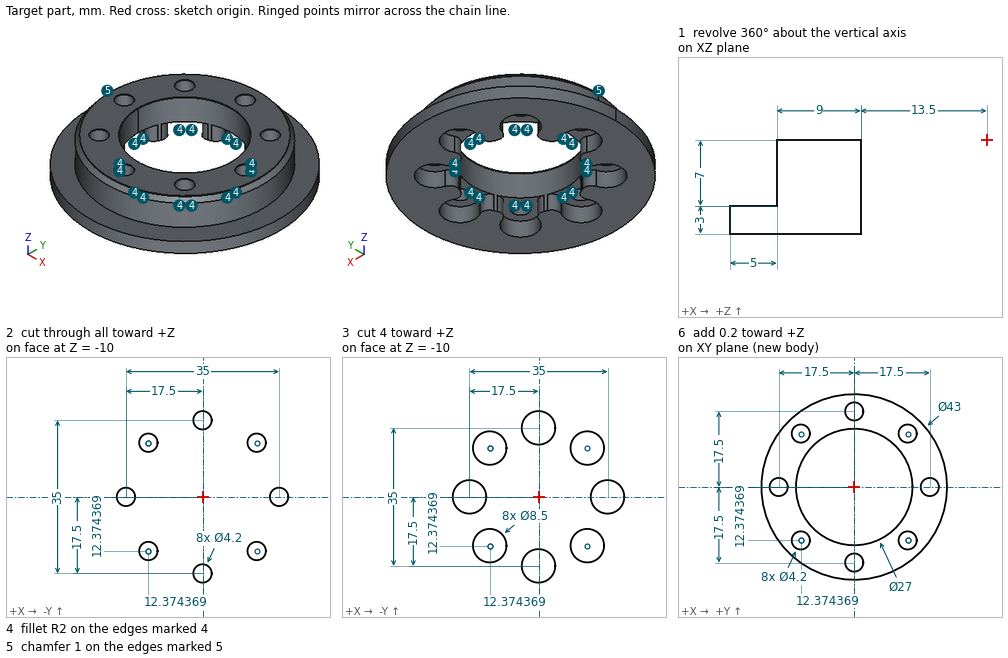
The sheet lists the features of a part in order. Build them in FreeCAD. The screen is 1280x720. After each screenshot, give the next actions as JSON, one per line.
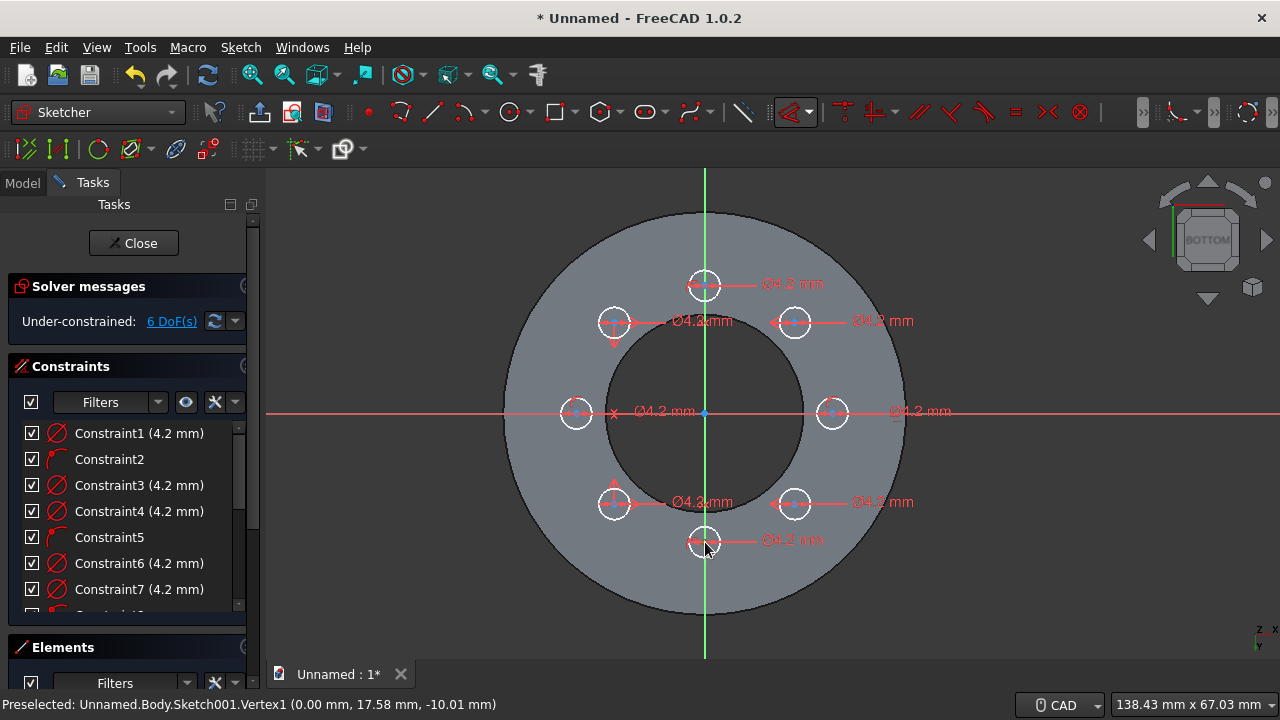
{"action": "left_click", "coordinate": [705, 286]}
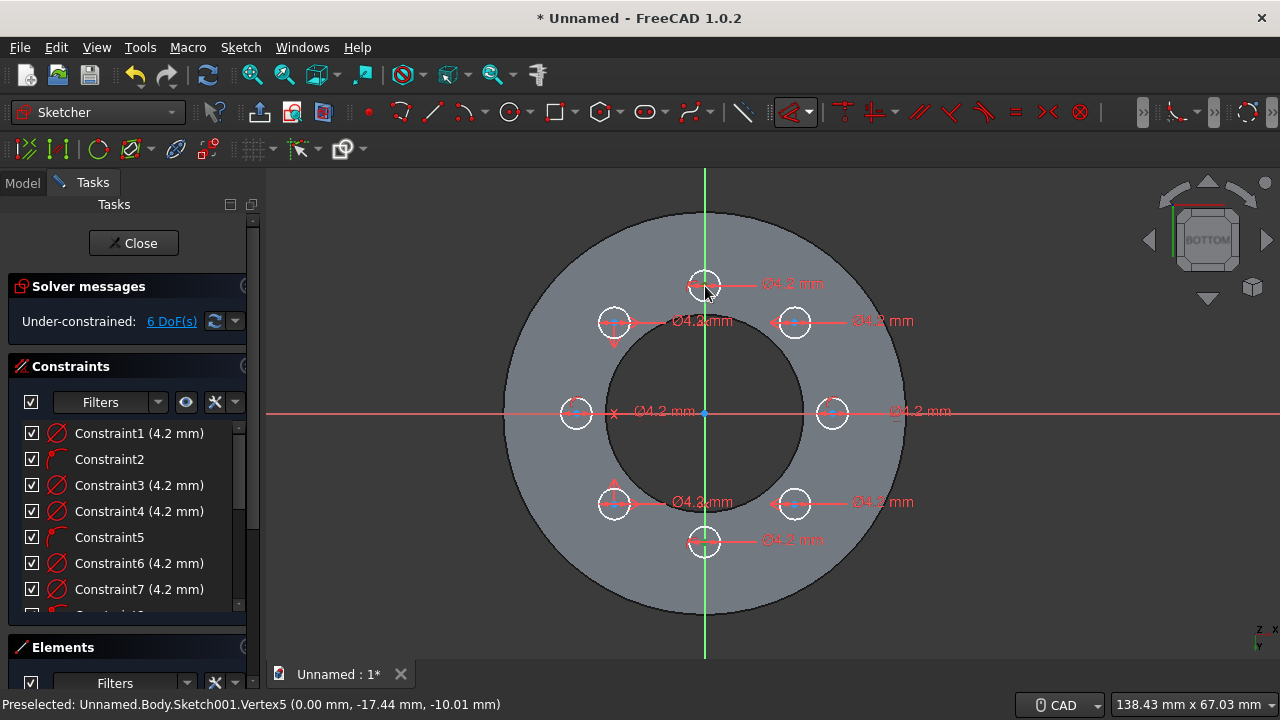
{"action": "key", "text": "i"}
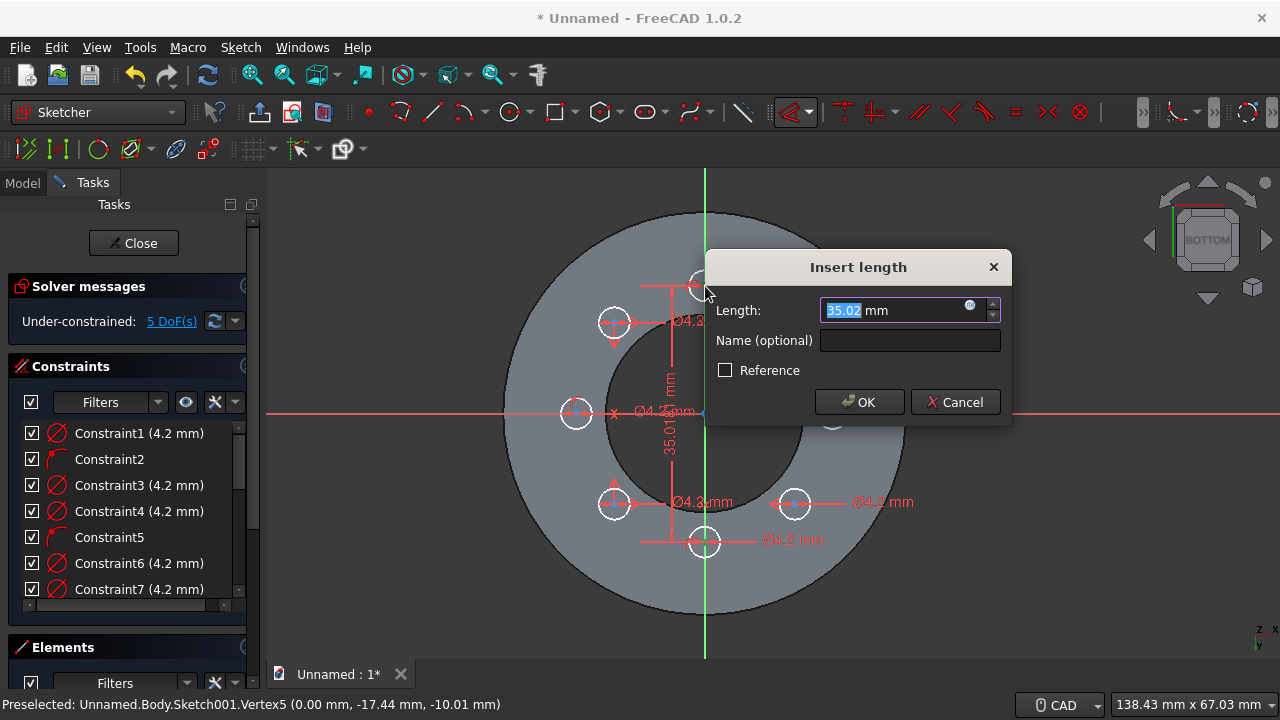
{"action": "type", "text": "35"}
{"action": "key", "text": "Return"}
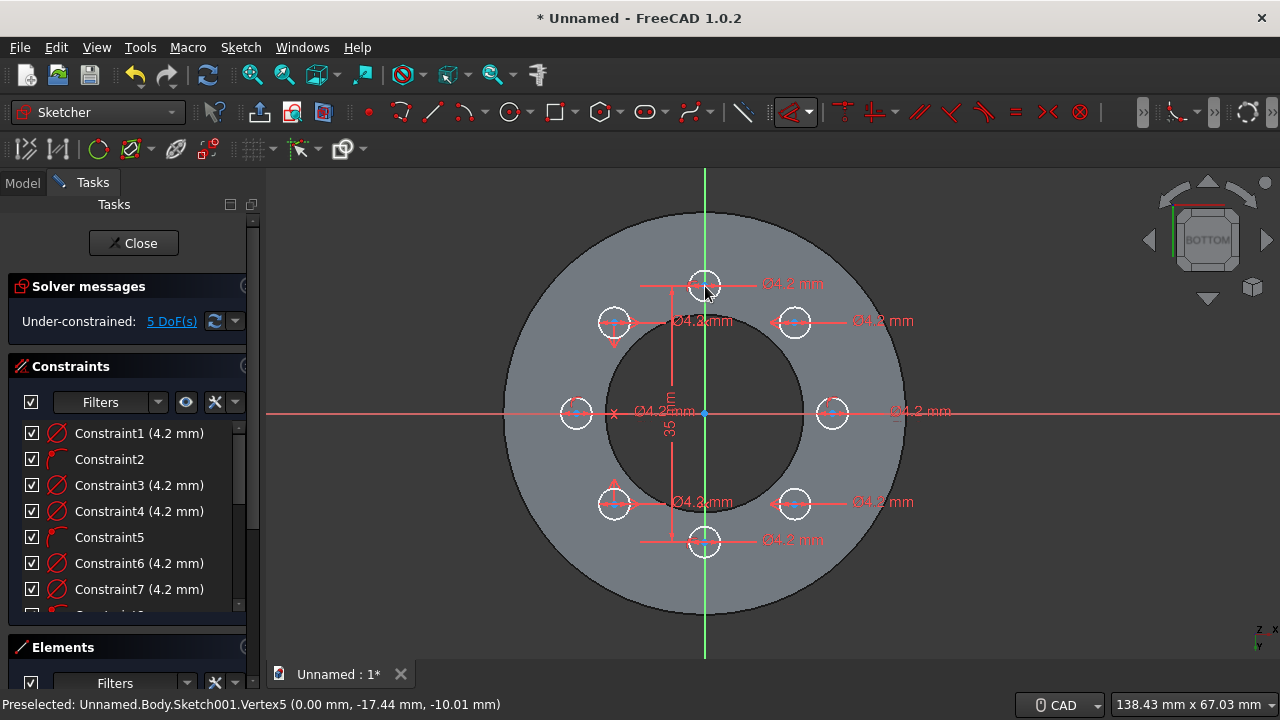
{"action": "left_click", "coordinate": [576, 414]}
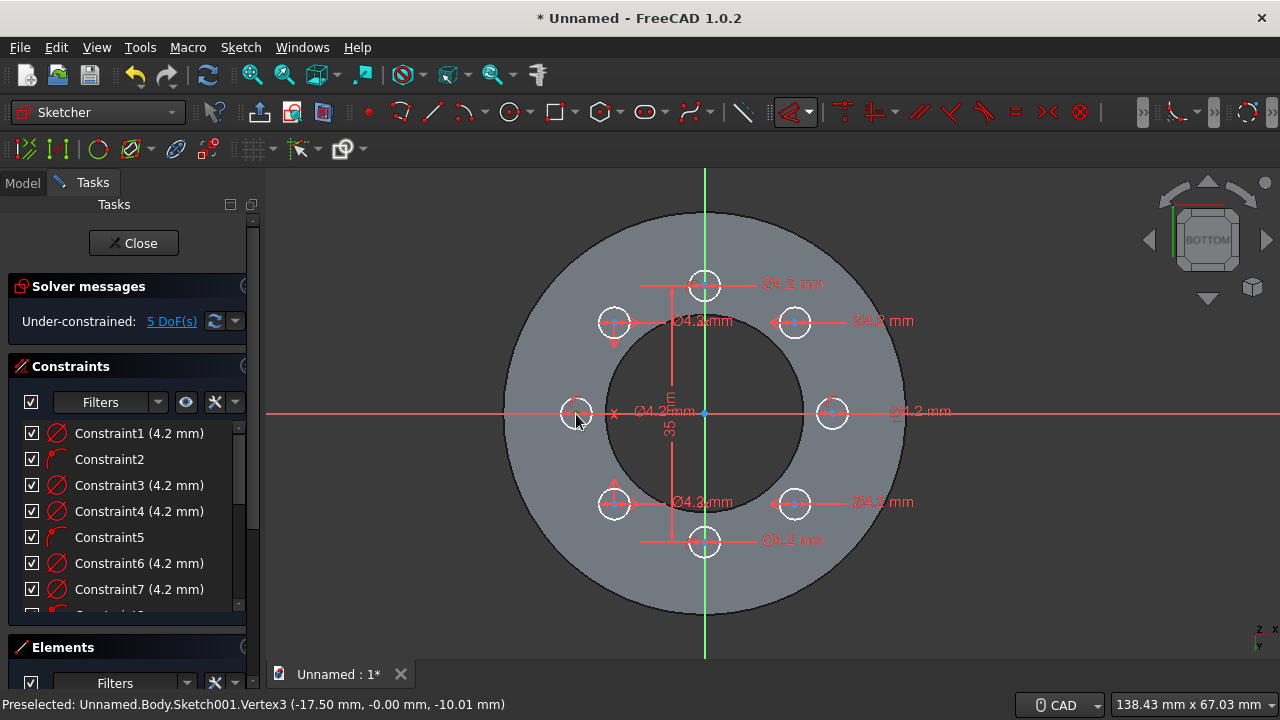
{"action": "left_click", "coordinate": [833, 414]}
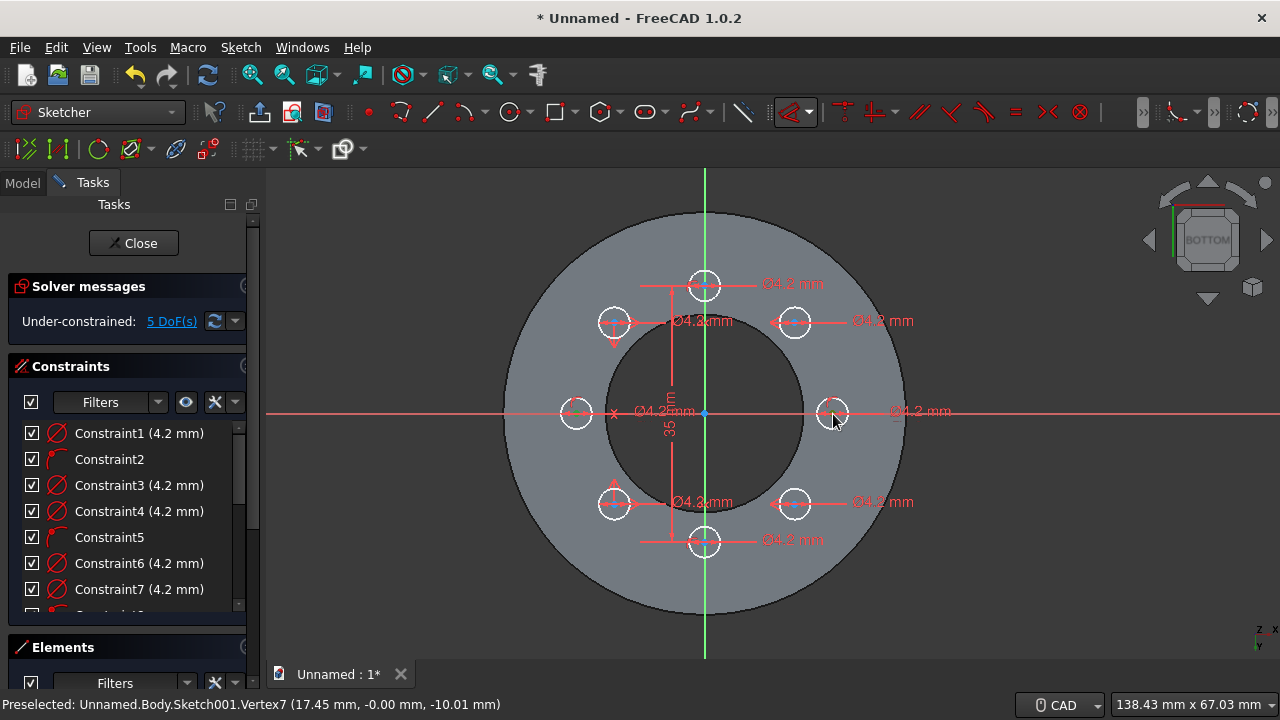
{"action": "key", "text": "l"}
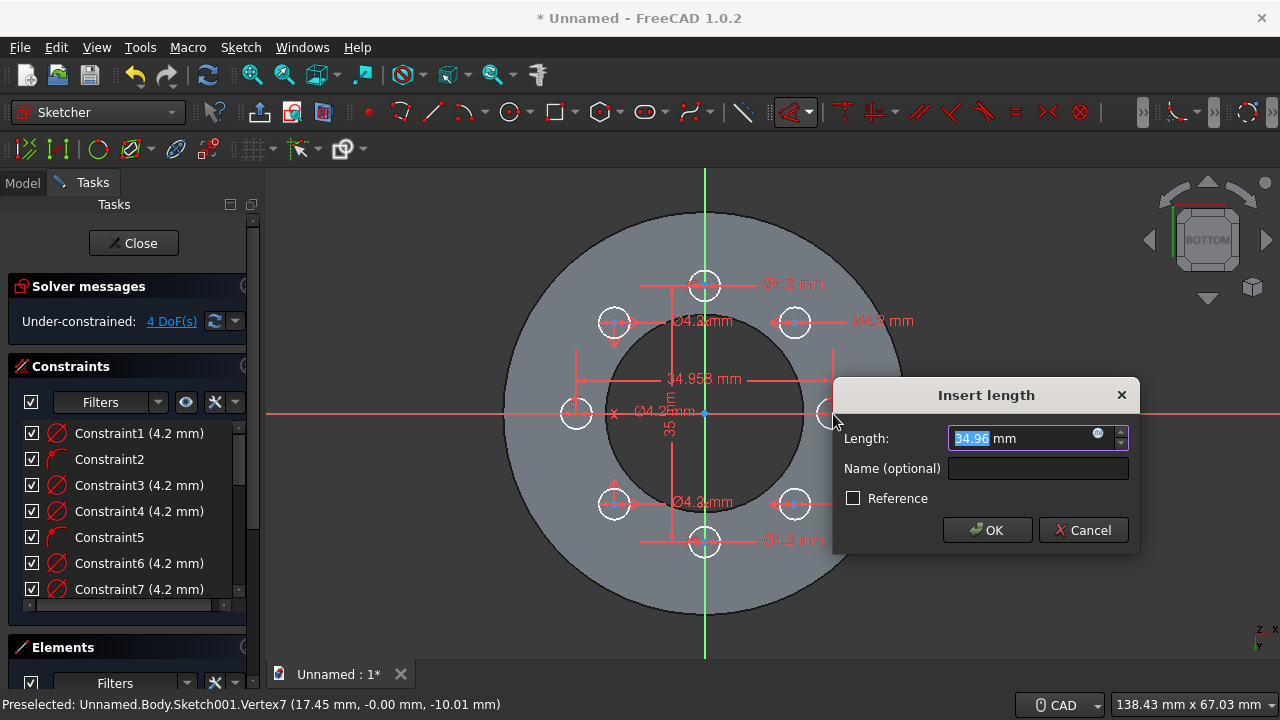
{"action": "type", "text": "35"}
{"action": "key", "text": "Return"}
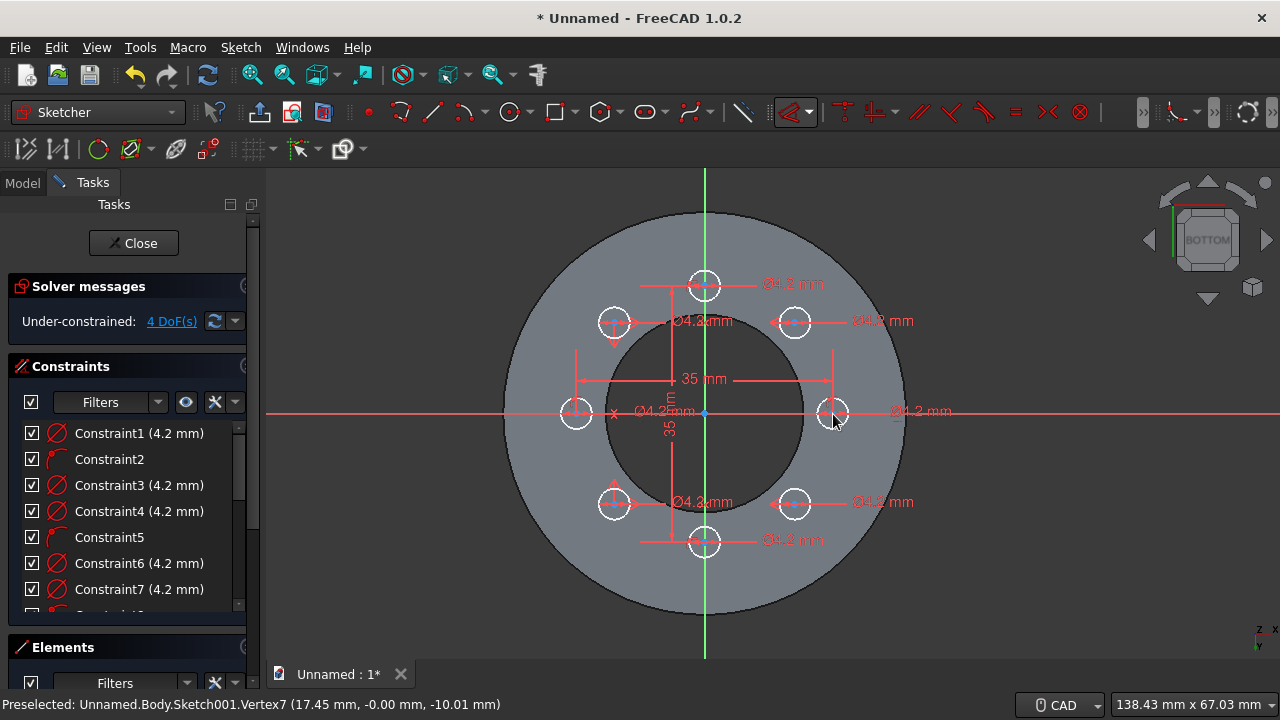
{"action": "left_click", "coordinate": [705, 542]}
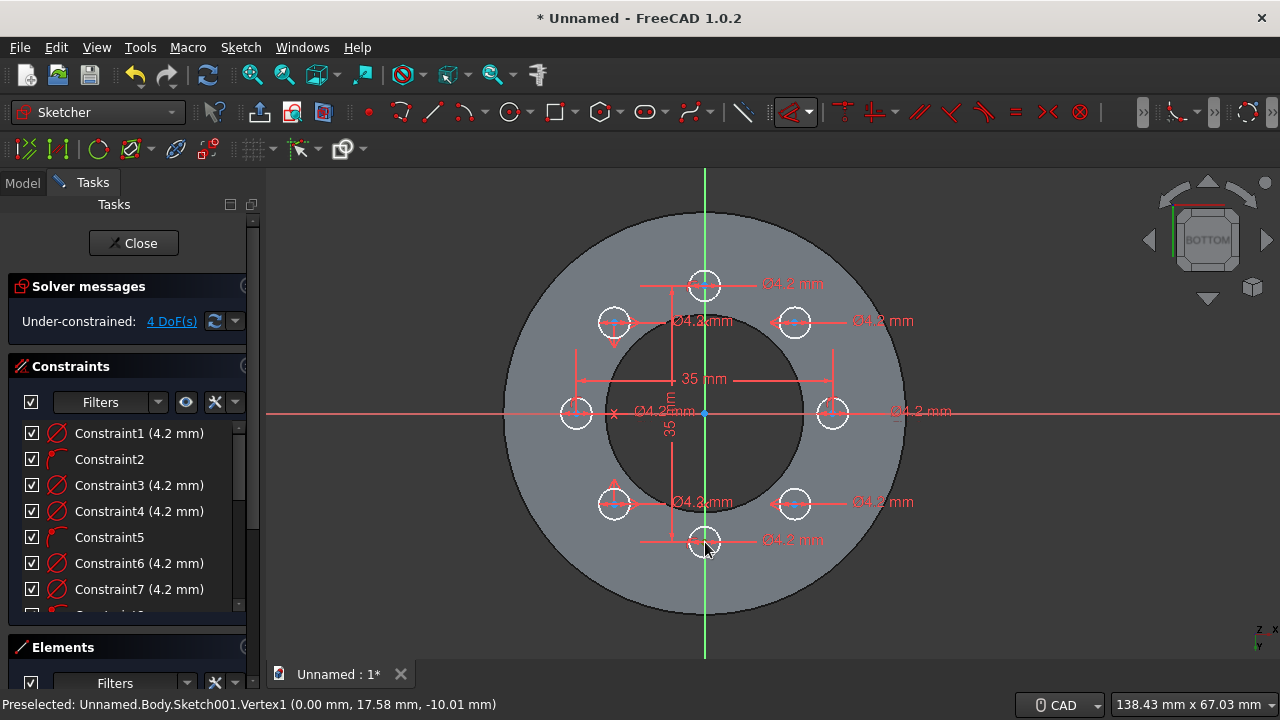
{"action": "key", "text": "i"}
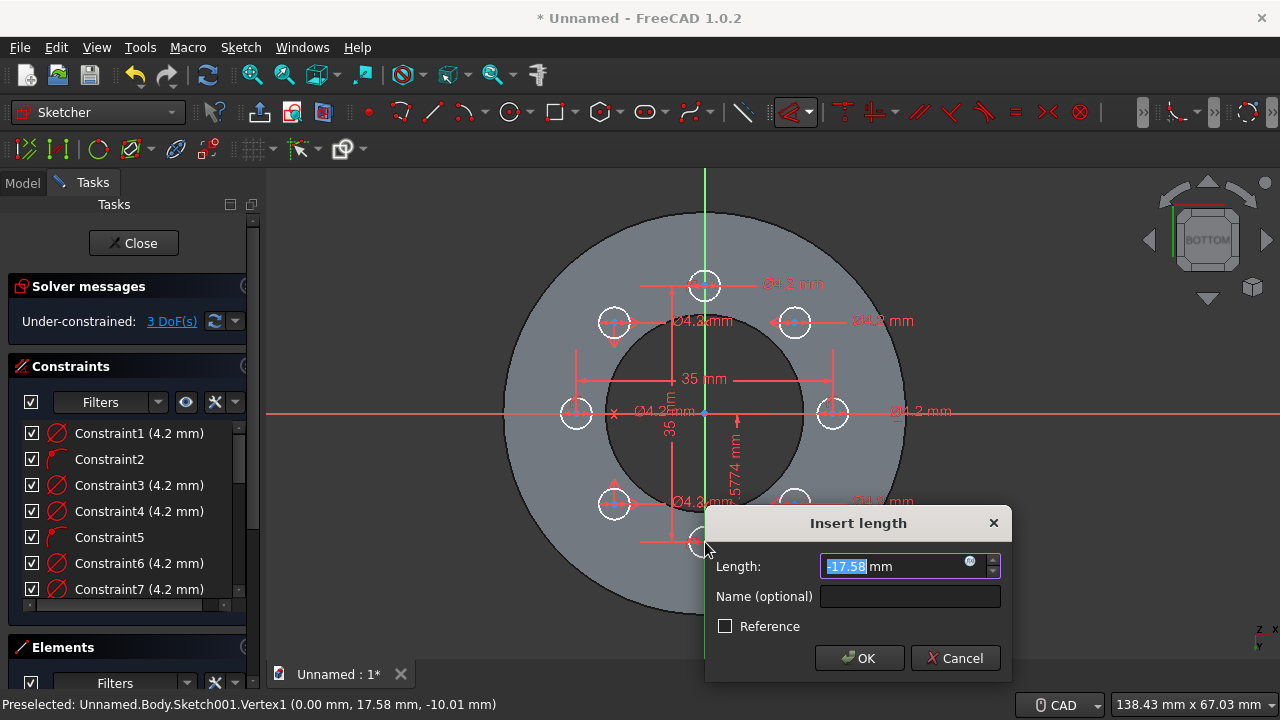
{"action": "type", "text": "-17.5"}
{"action": "key", "text": "Return"}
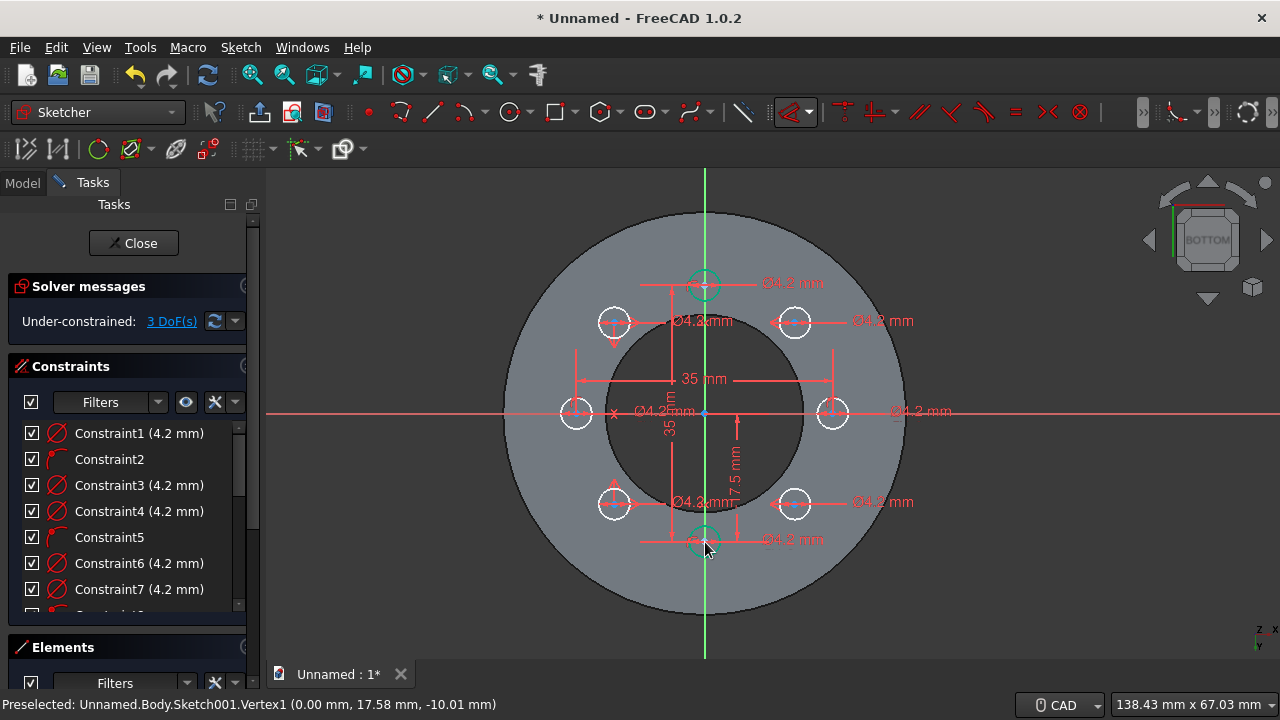
{"action": "left_click", "coordinate": [576, 414]}